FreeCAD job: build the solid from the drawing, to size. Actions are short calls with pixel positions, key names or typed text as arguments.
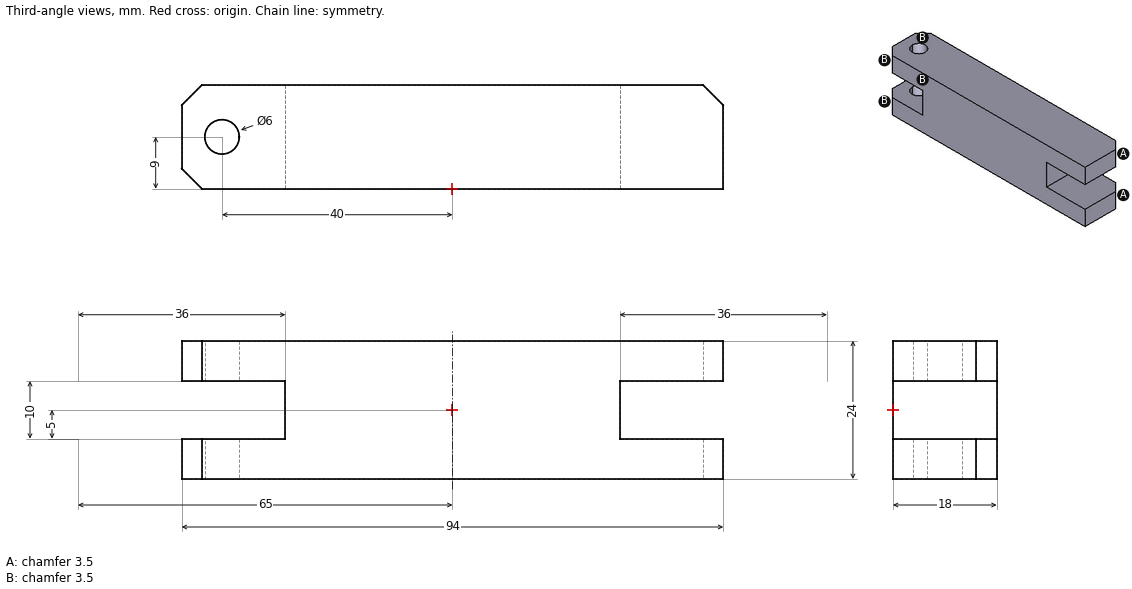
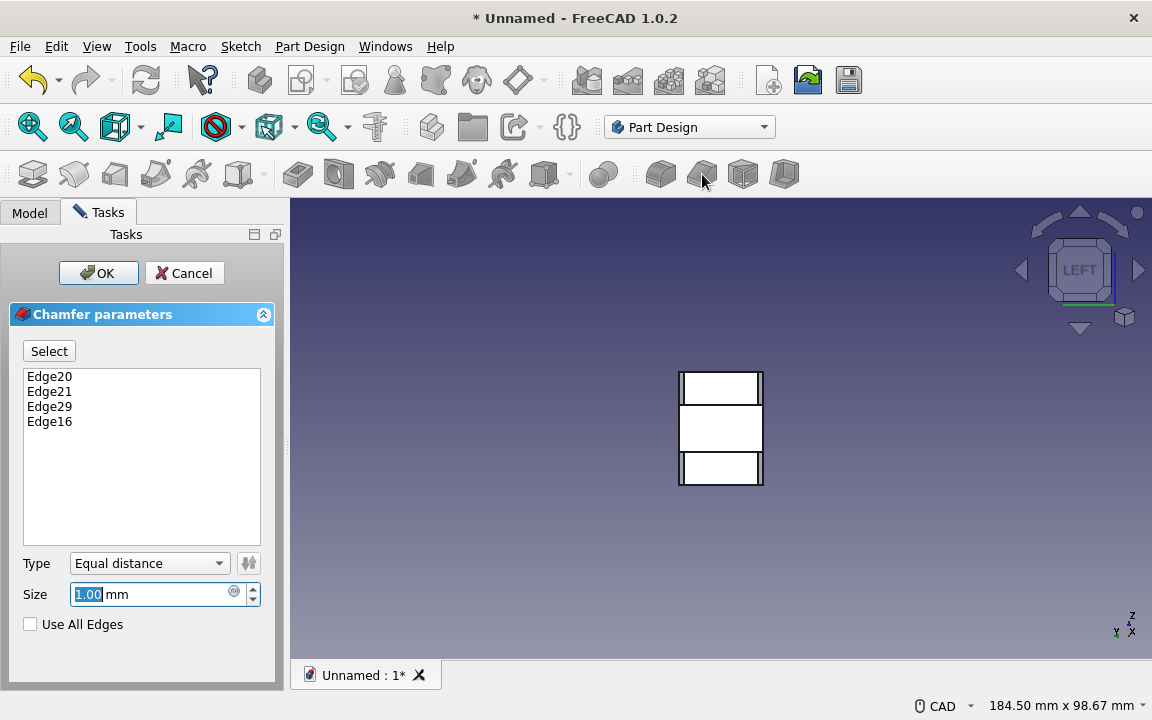
text(3.5)
key(Tab)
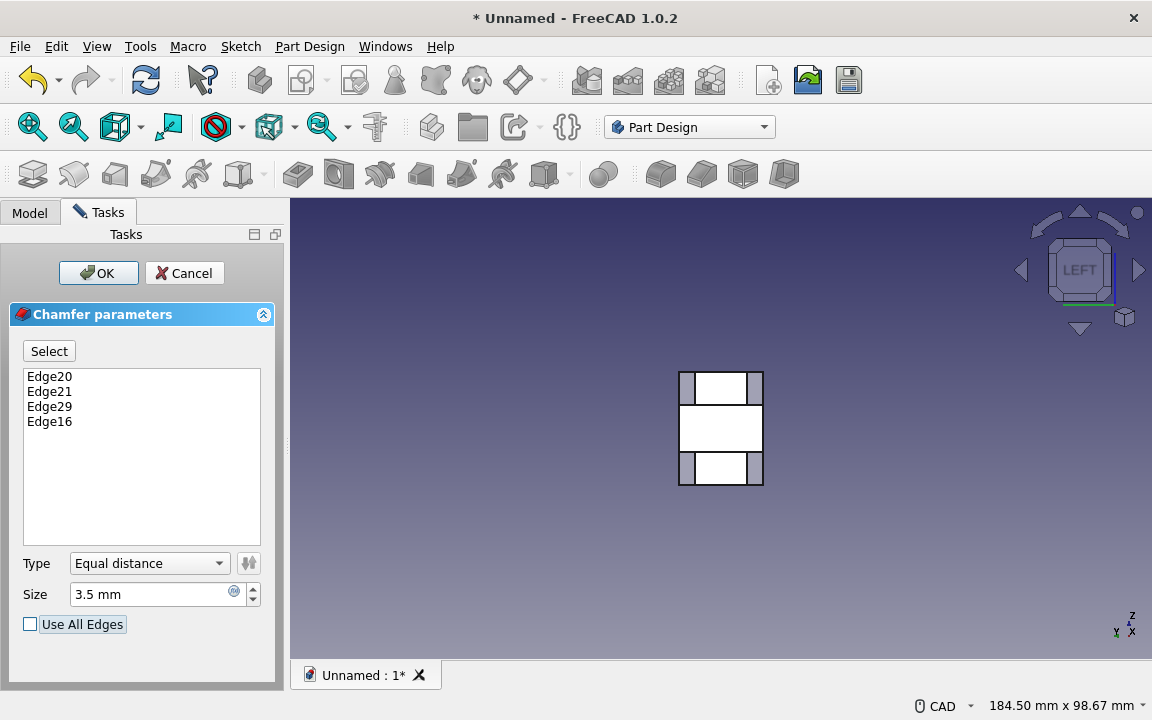
click(99, 273)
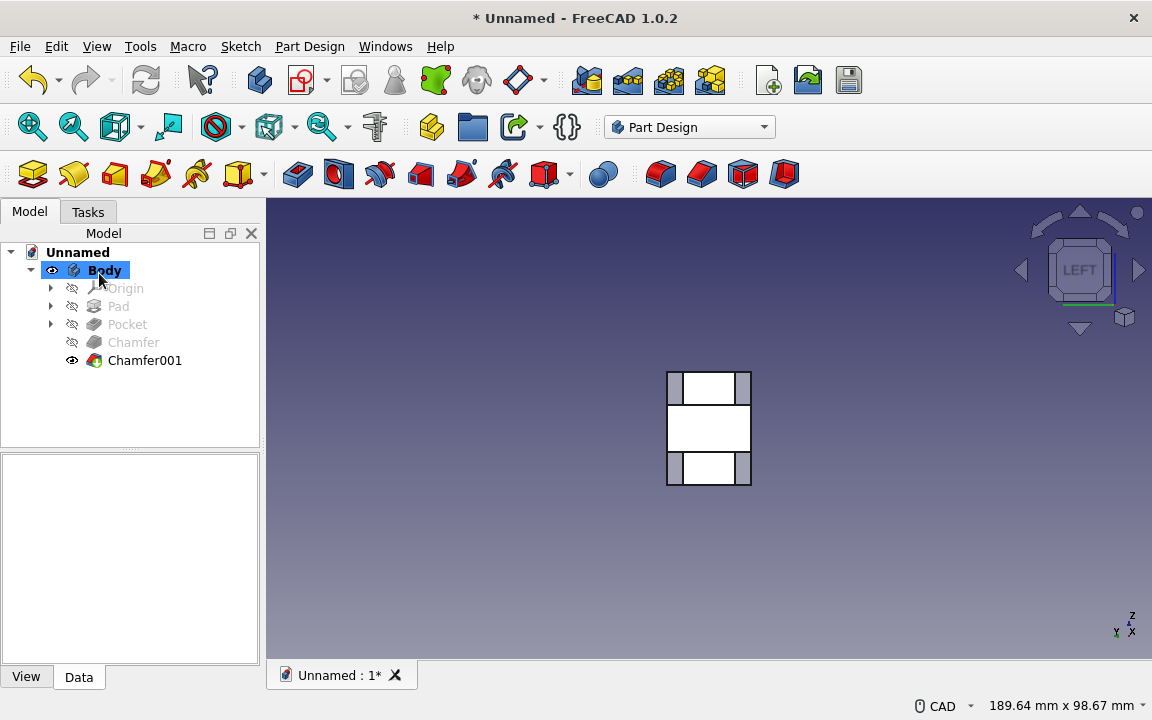
key(v)
key(f)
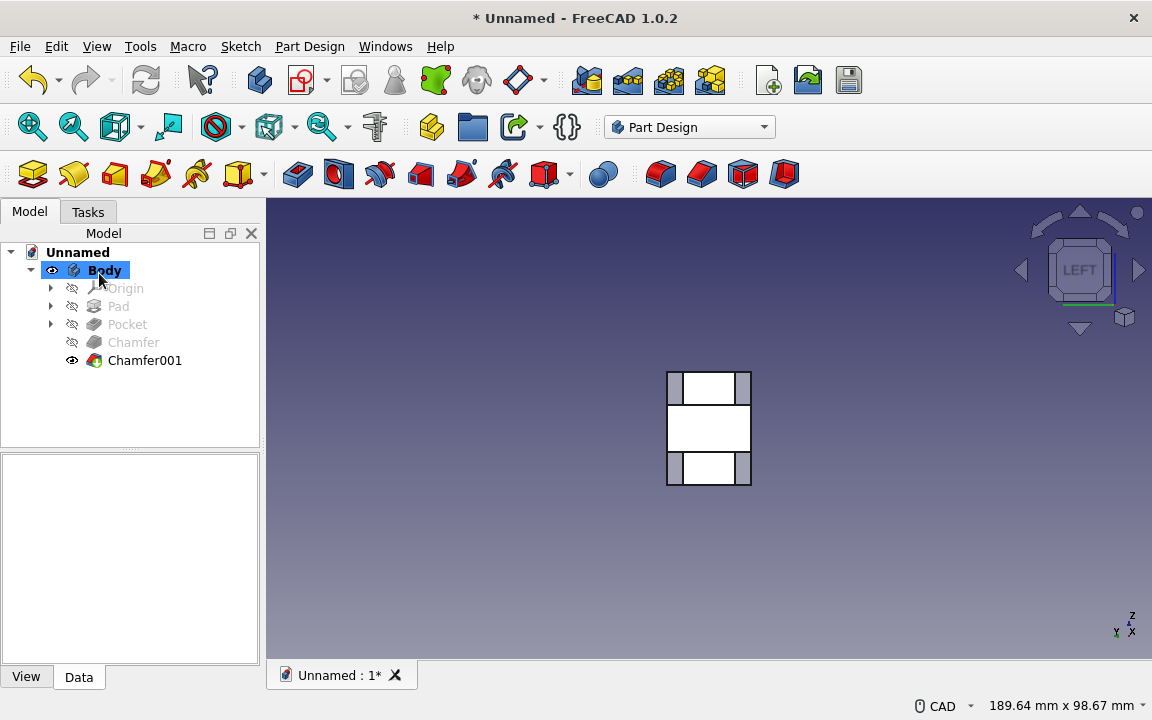
key(0)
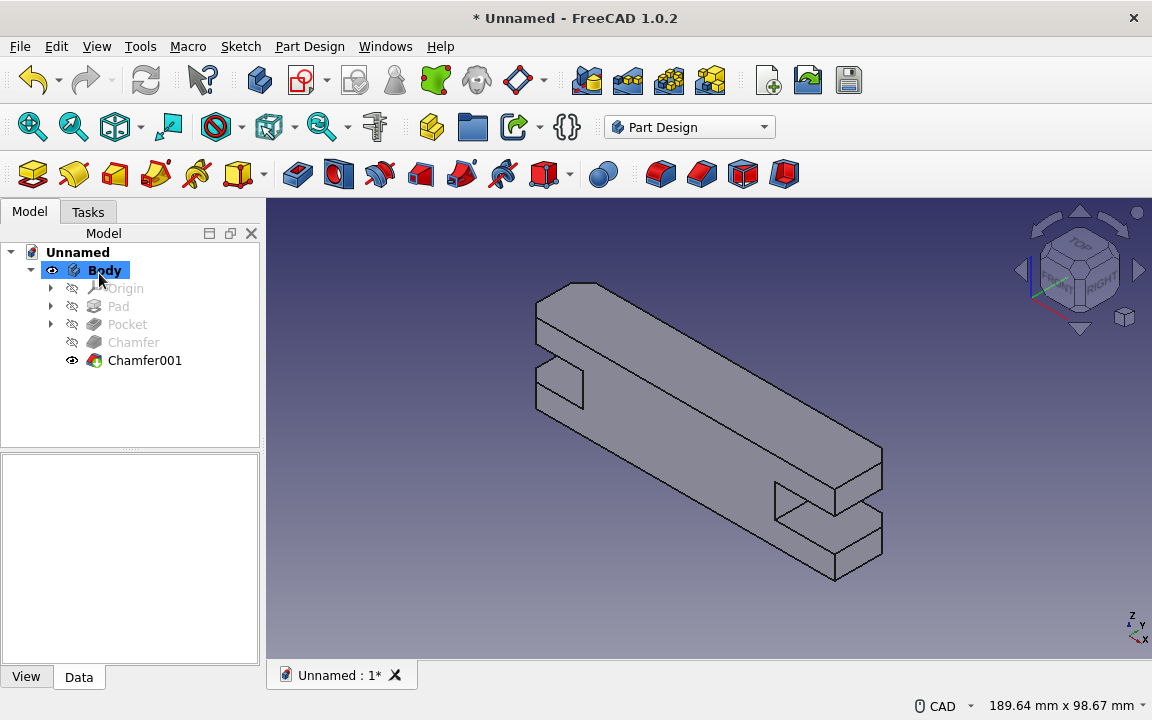
click(798, 433)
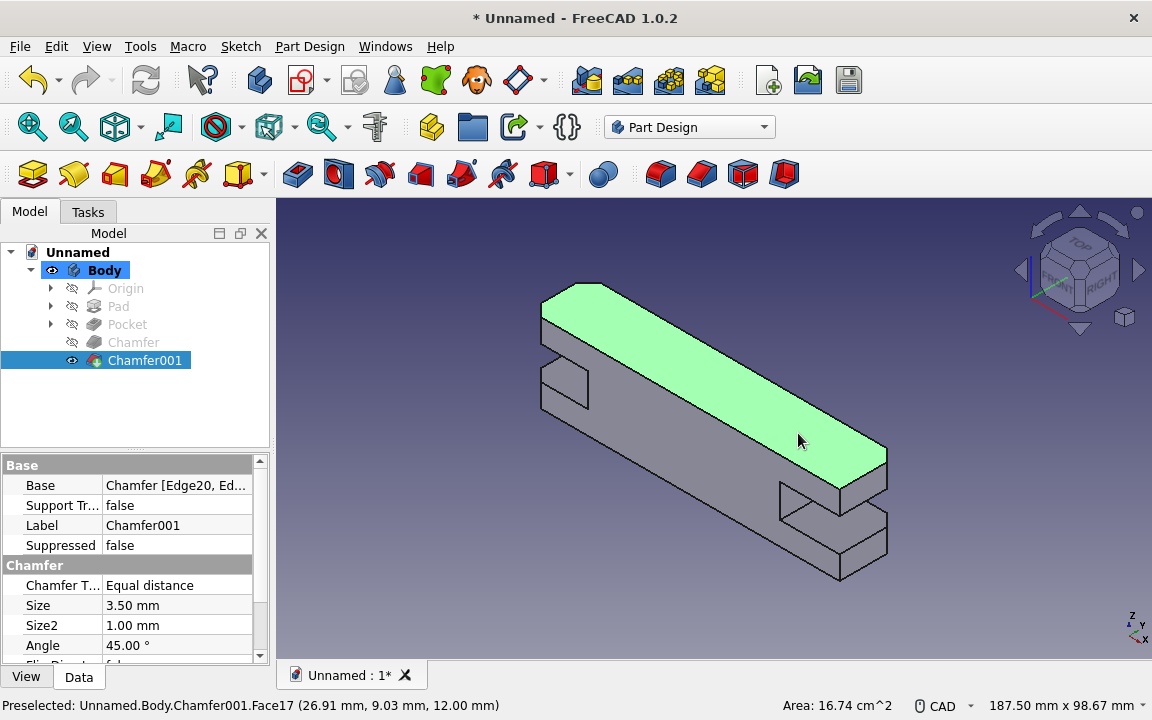
click(300, 80)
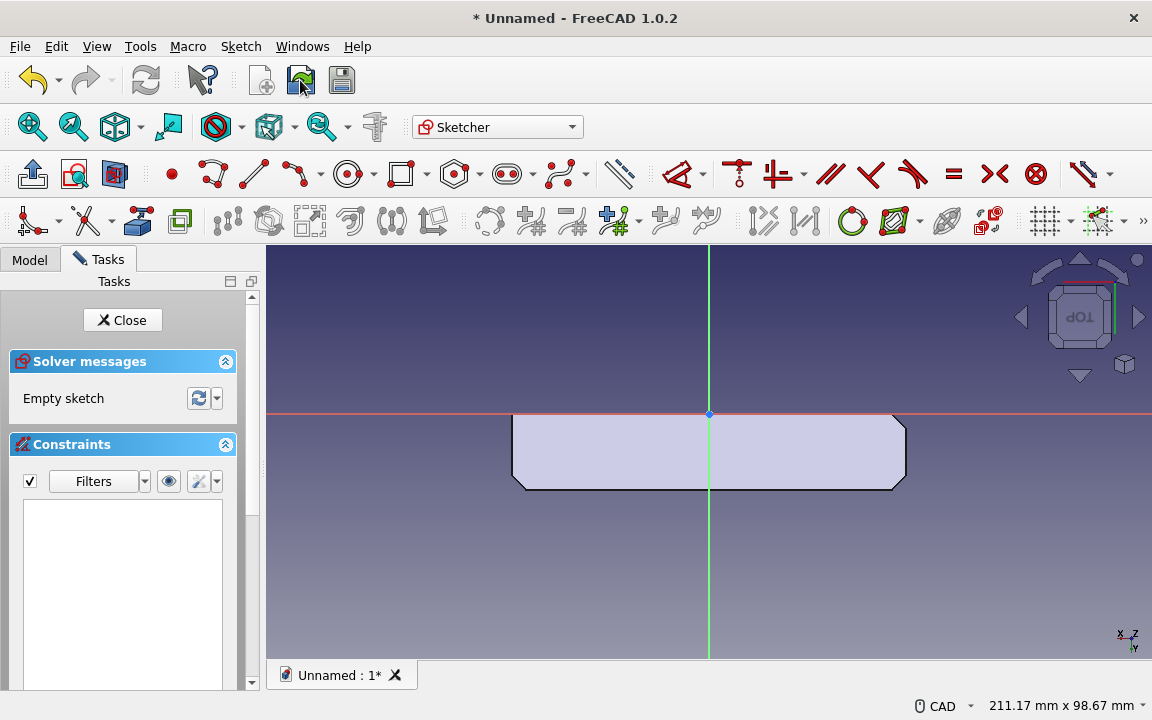
scroll(900, 452, up, 12)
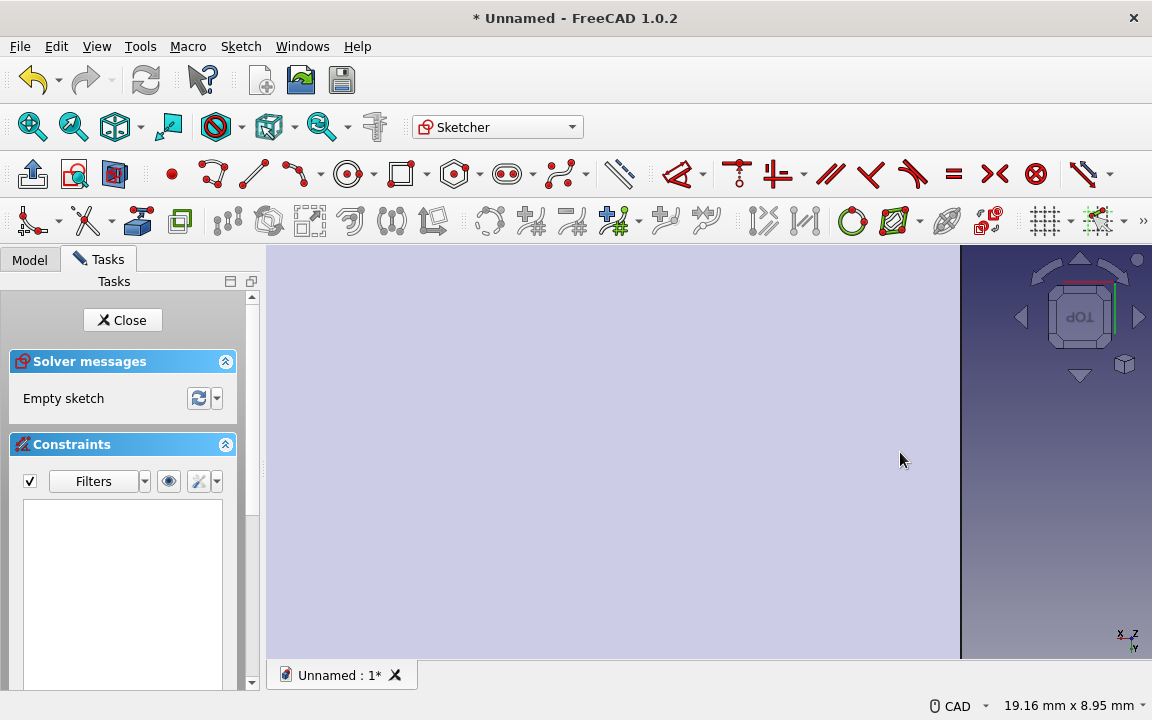
click(348, 174)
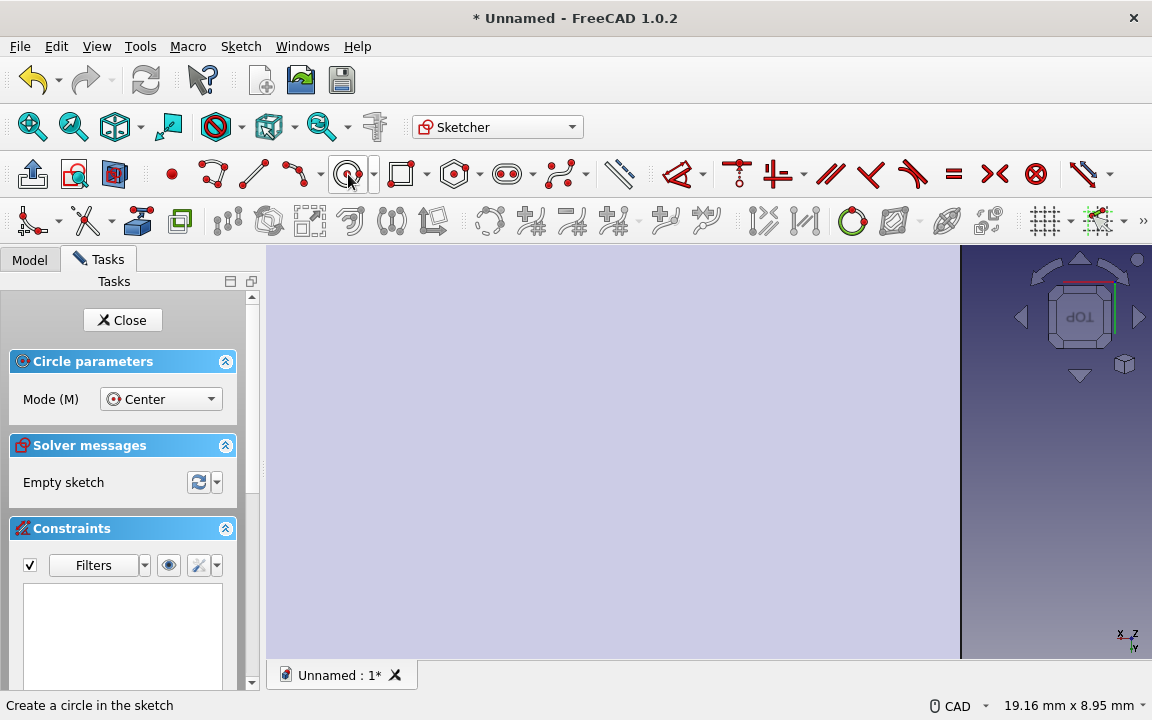
click(637, 447)
move(736, 349)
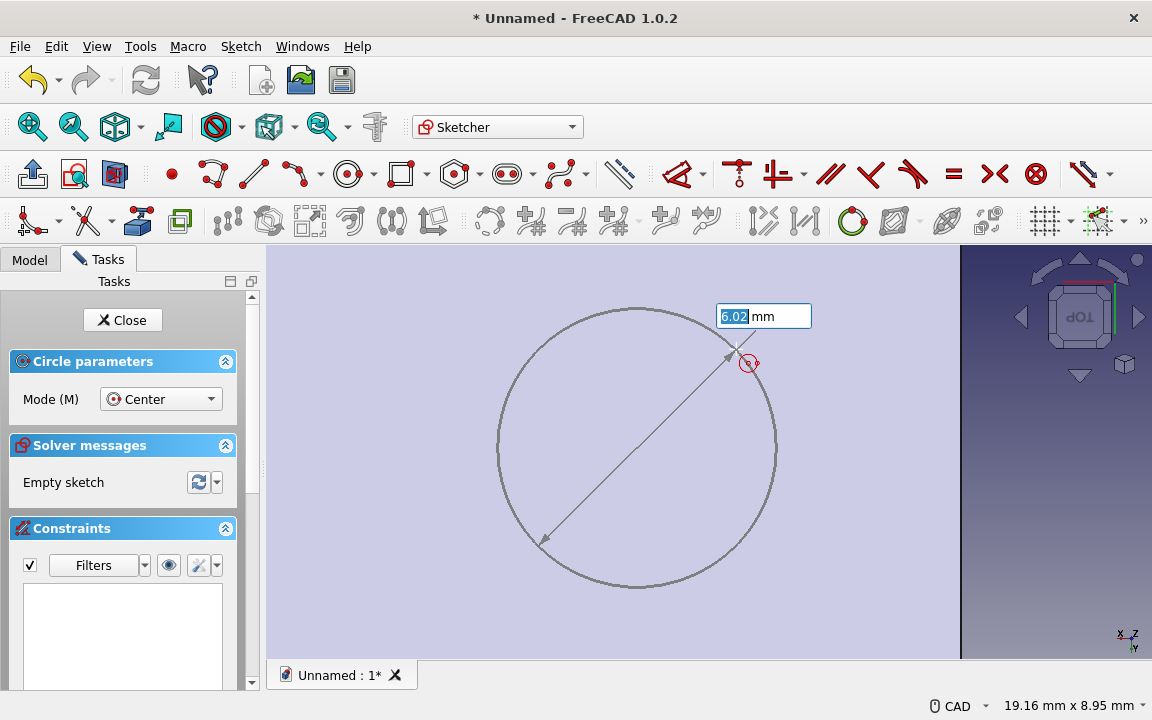
text(6)
key(Return)
key(Escape)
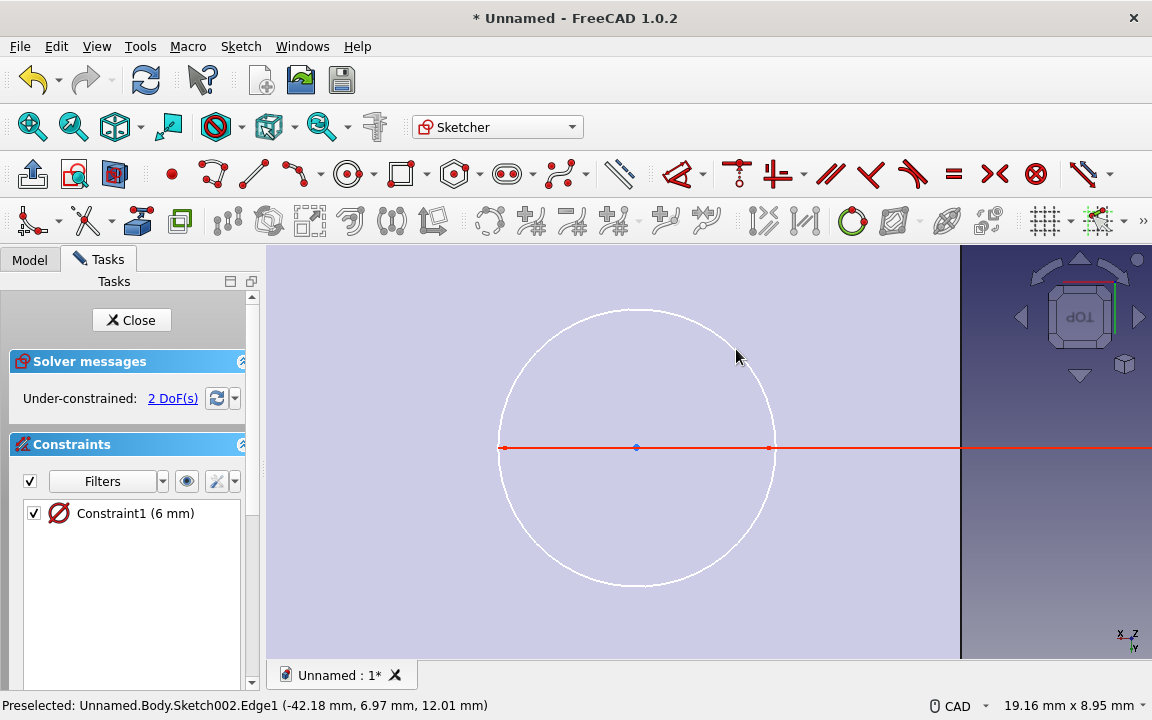
click(676, 174)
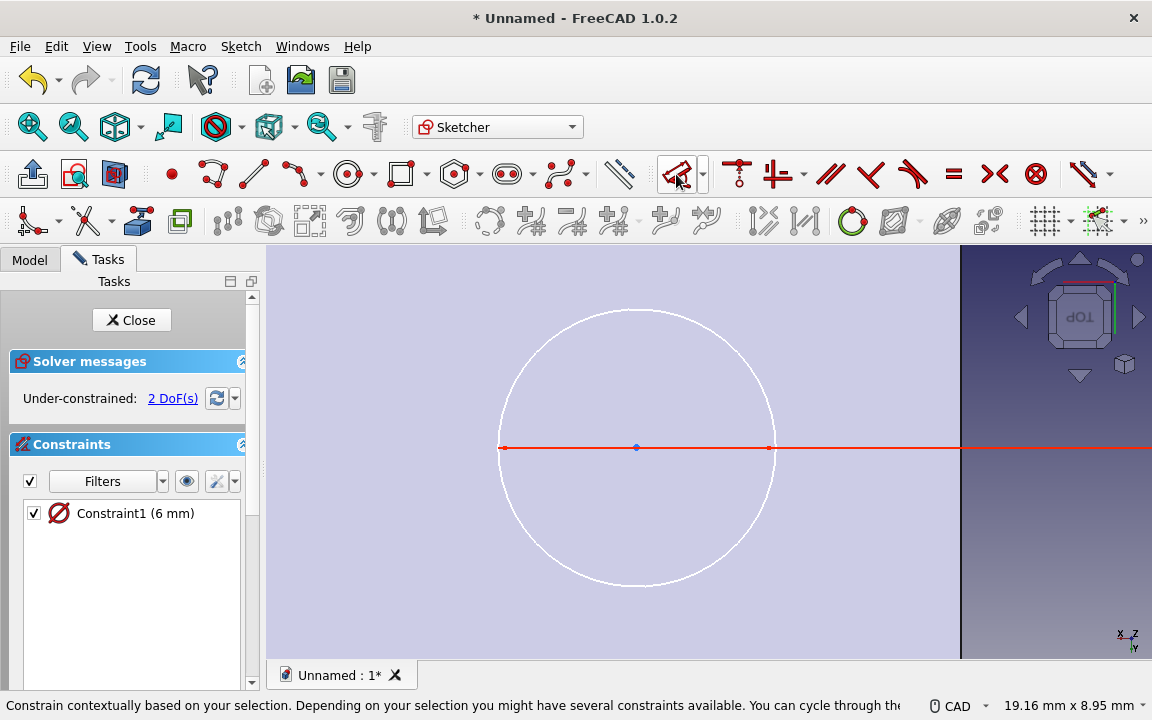
click(637, 448)
click(671, 360)